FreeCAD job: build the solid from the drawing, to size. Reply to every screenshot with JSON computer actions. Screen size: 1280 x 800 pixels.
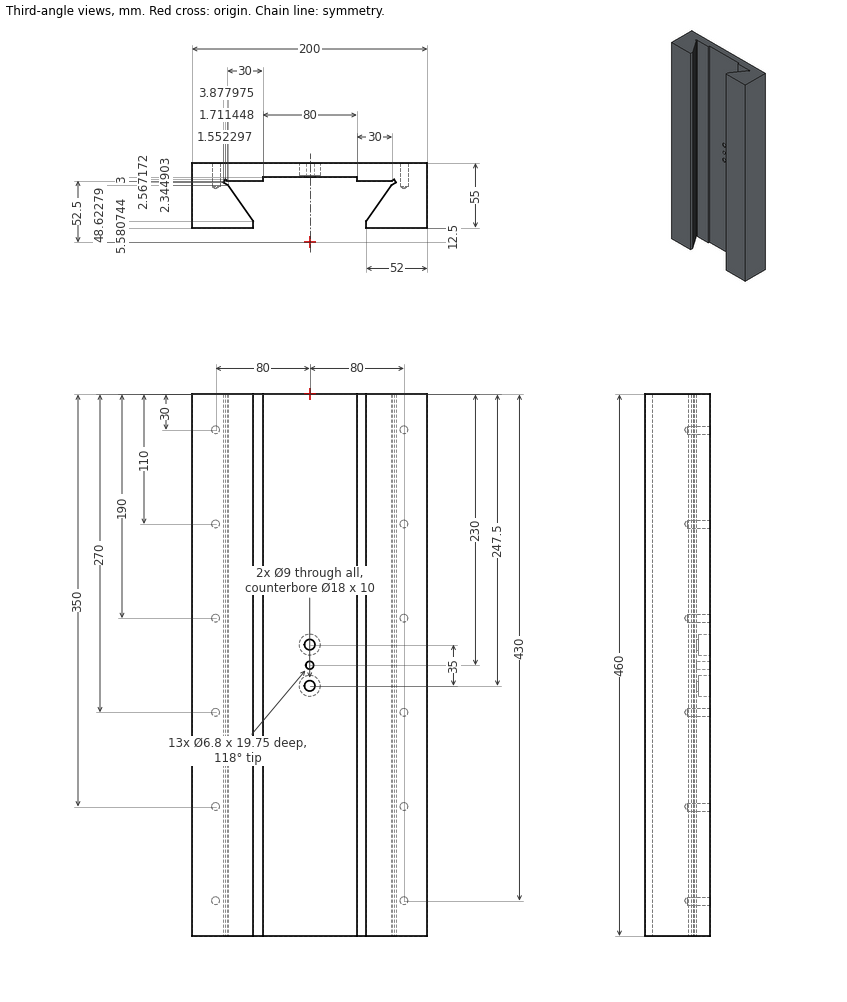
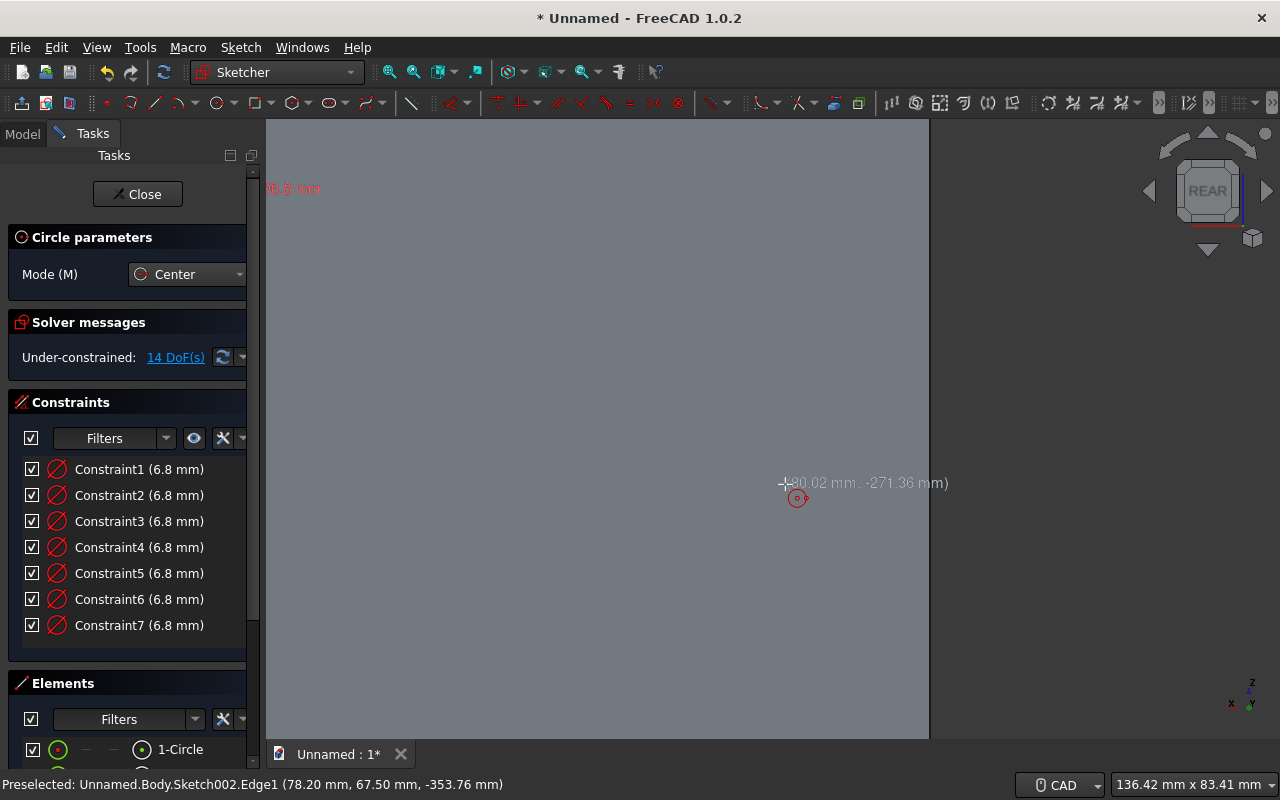
{"action": "scroll", "coordinate": [786, 483], "scroll_direction": "down", "scroll_amount": 10}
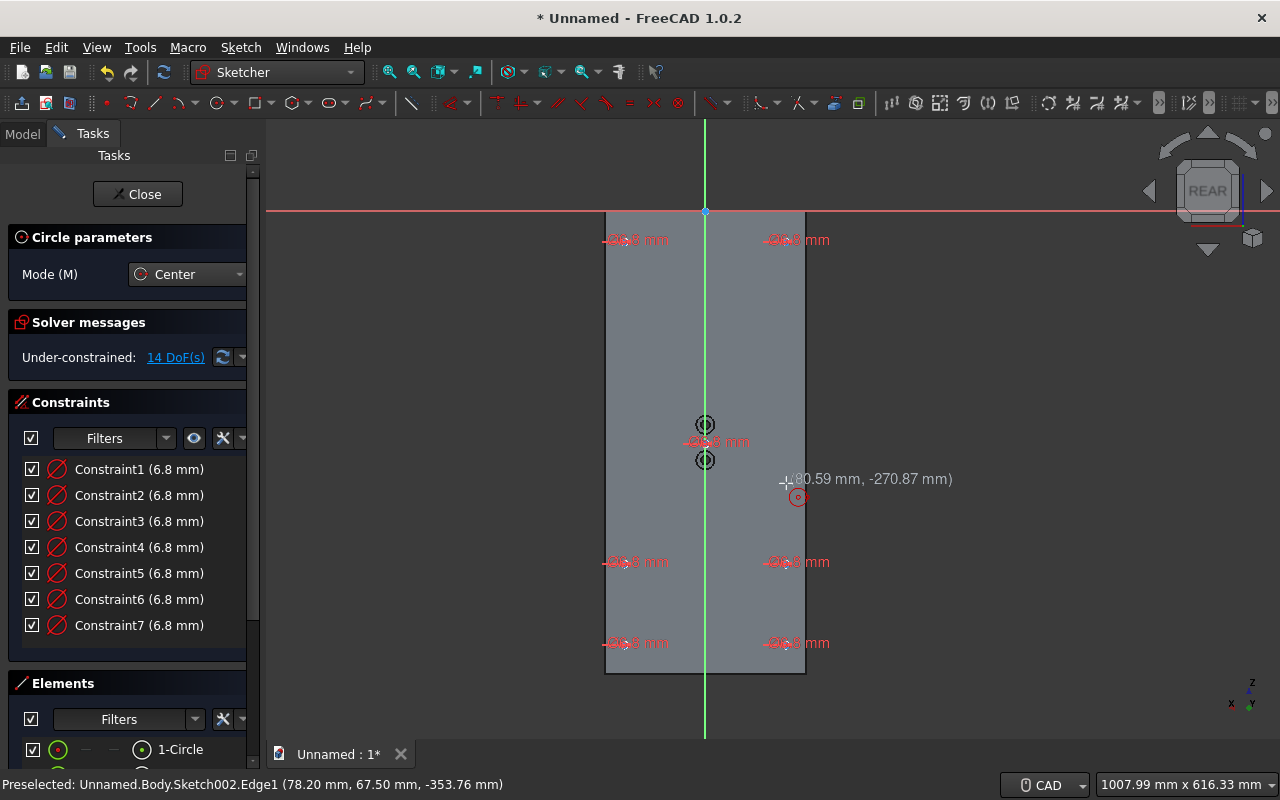
{"action": "left_click", "coordinate": [786, 483]}
{"action": "mouse_move", "coordinate": [788, 480]}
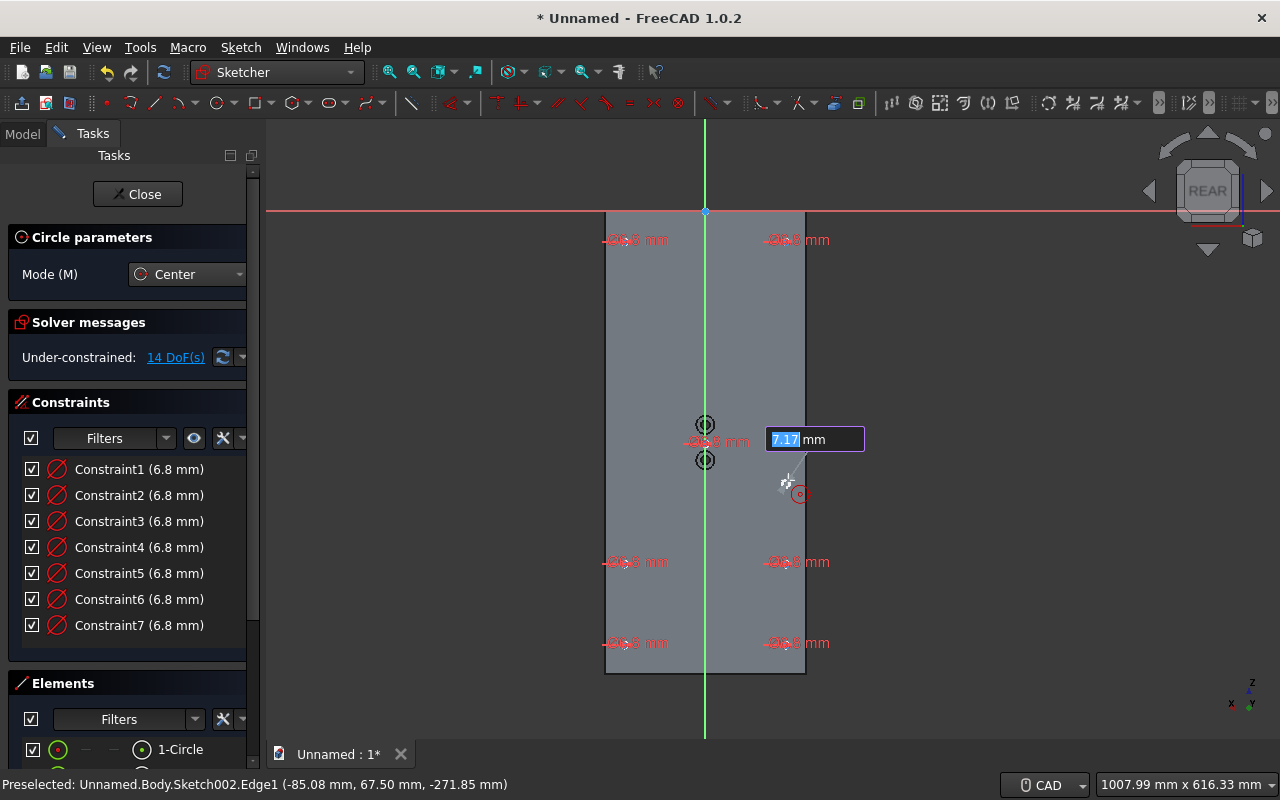
{"action": "type", "text": "6.8"}
{"action": "key", "text": "Return"}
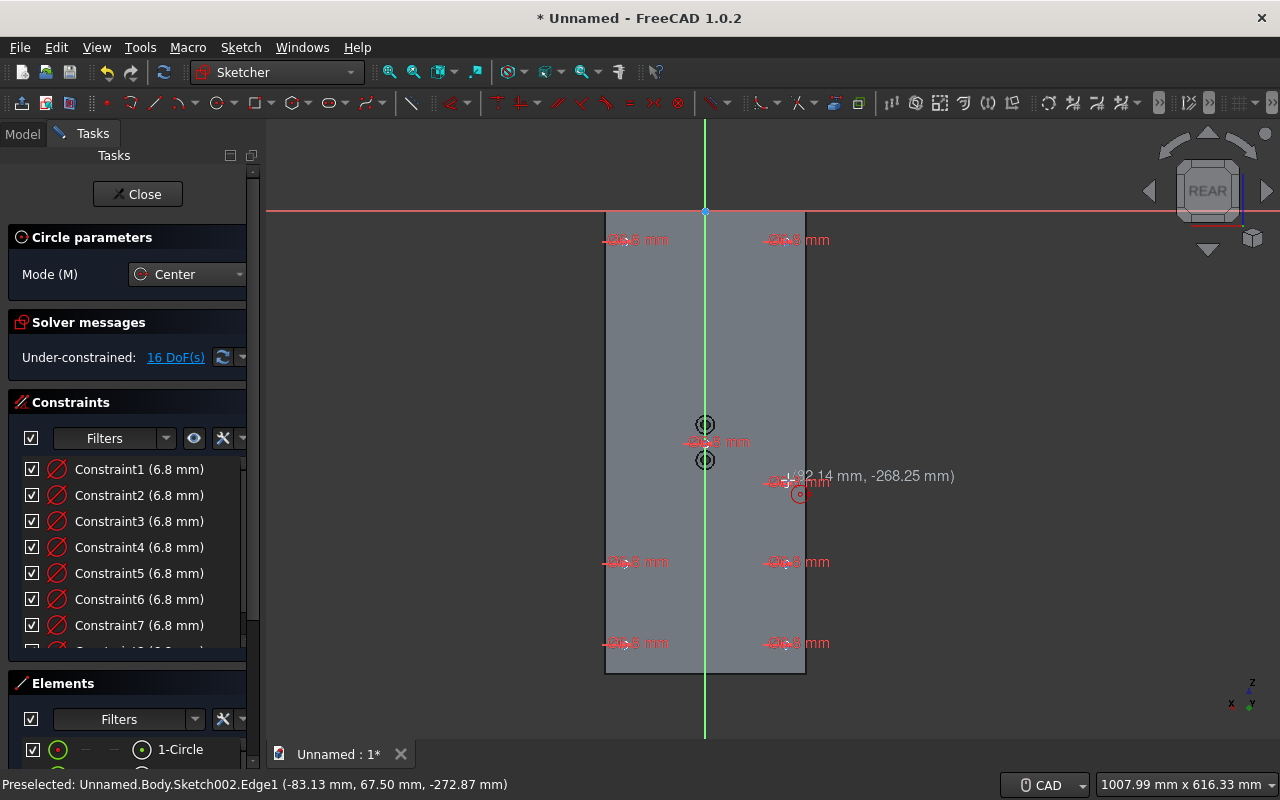
{"action": "scroll", "coordinate": [625, 483], "scroll_direction": "up", "scroll_amount": 10}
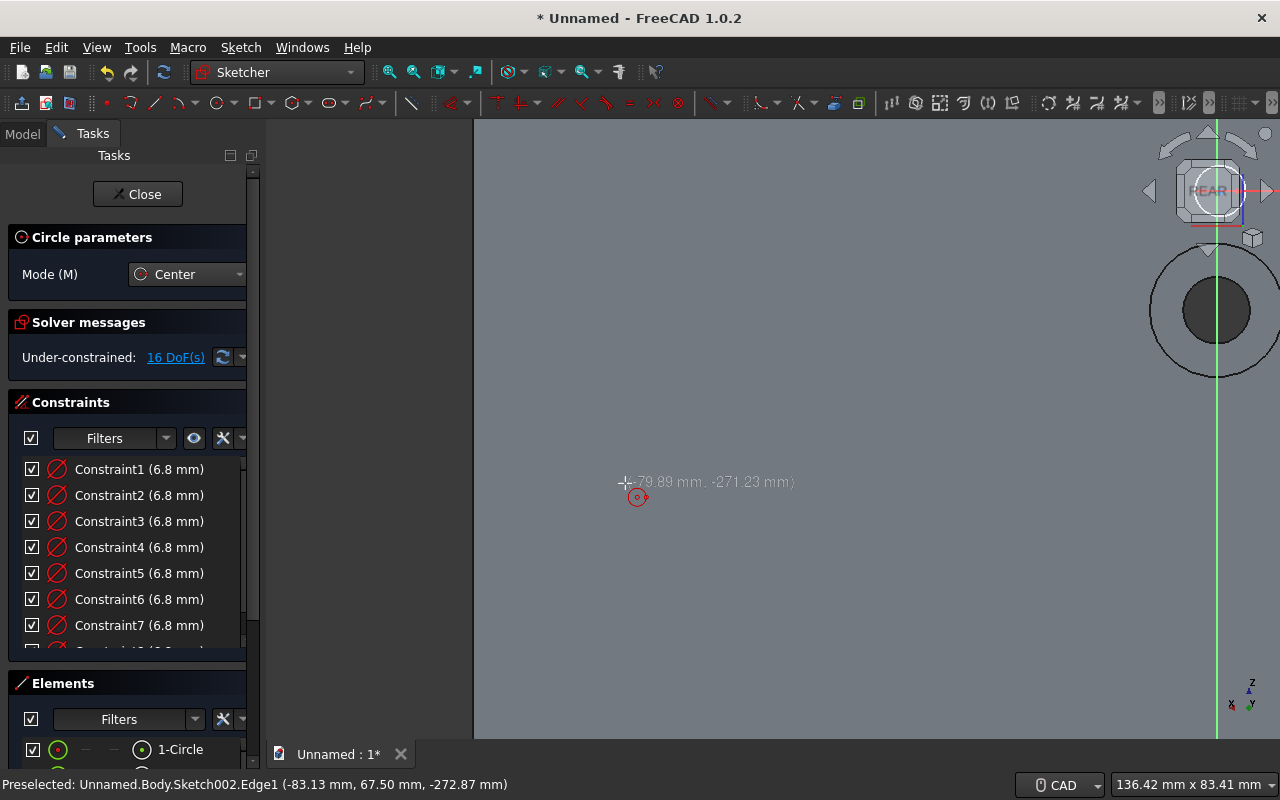
{"action": "scroll", "coordinate": [624, 483], "scroll_direction": "down", "scroll_amount": 10}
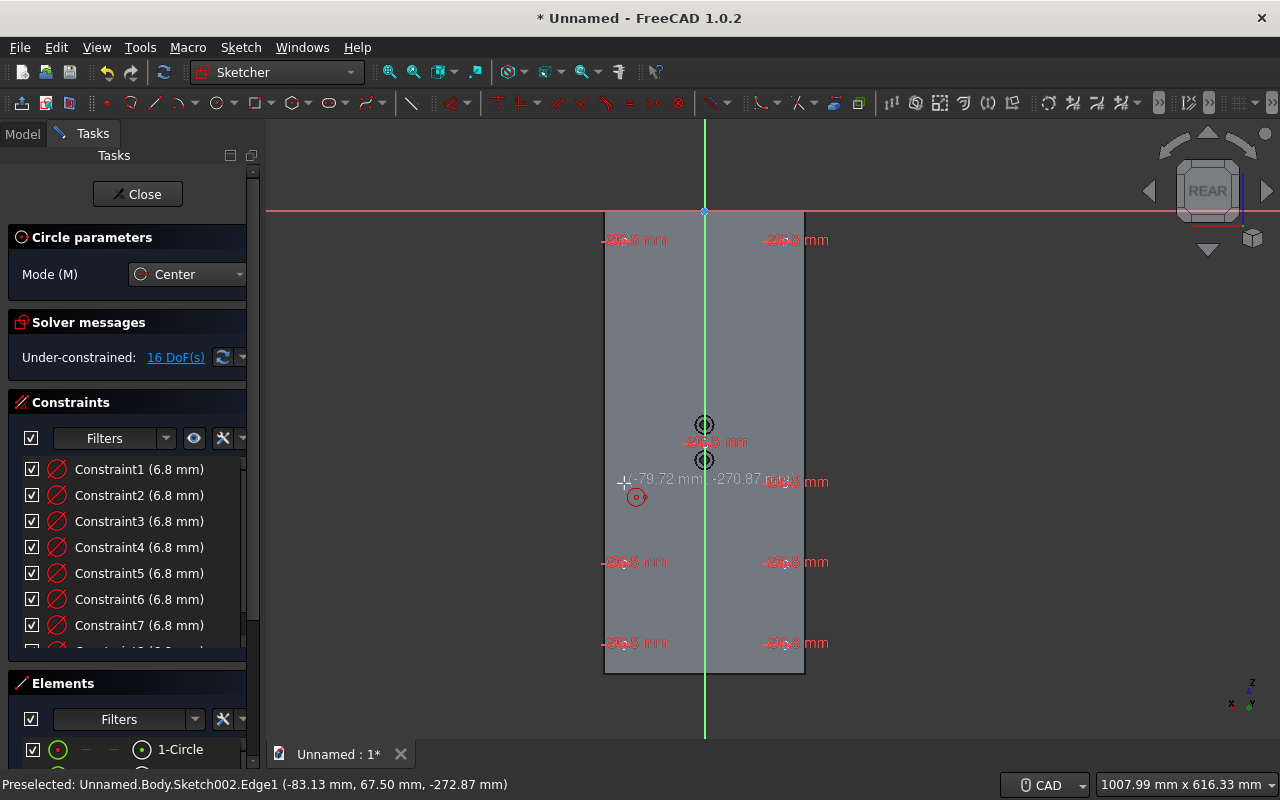
{"action": "left_click", "coordinate": [624, 483]}
{"action": "mouse_move", "coordinate": [626, 480]}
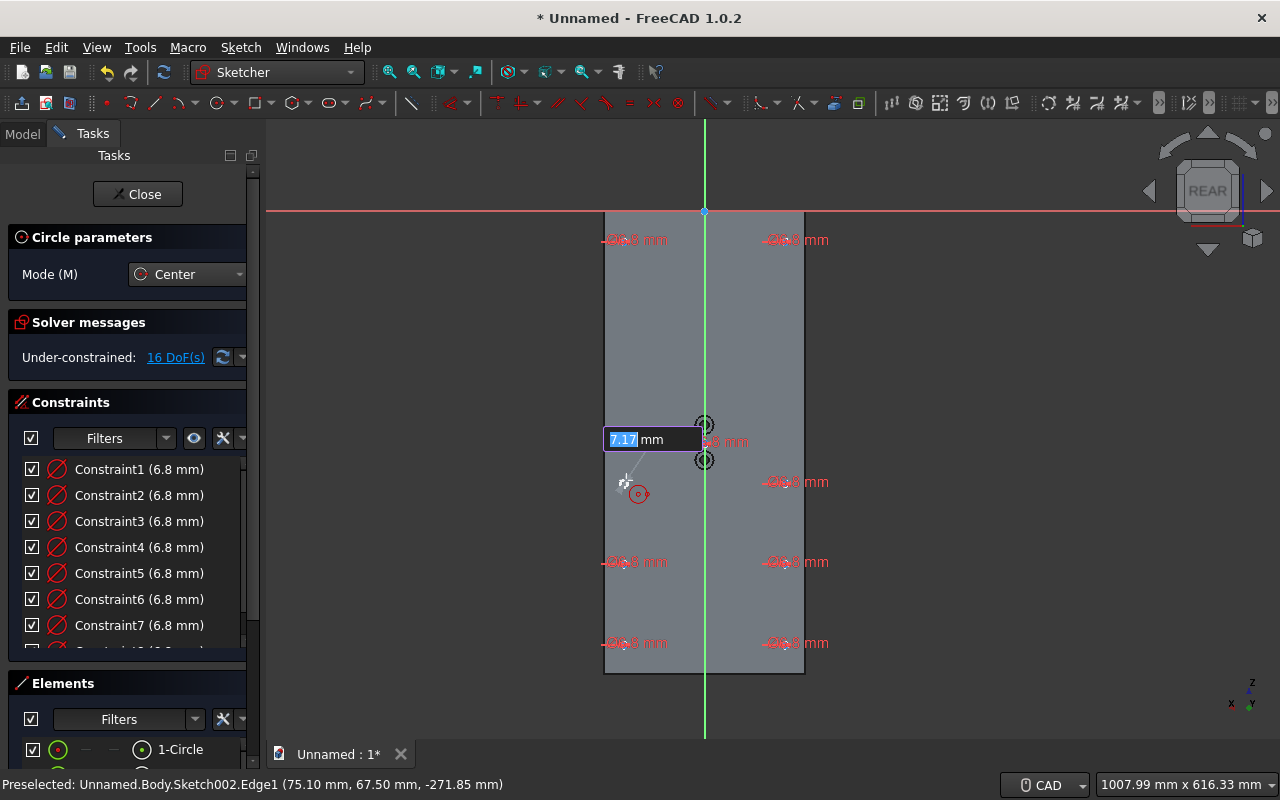
{"action": "type", "text": "6.8"}
{"action": "key", "text": "Return"}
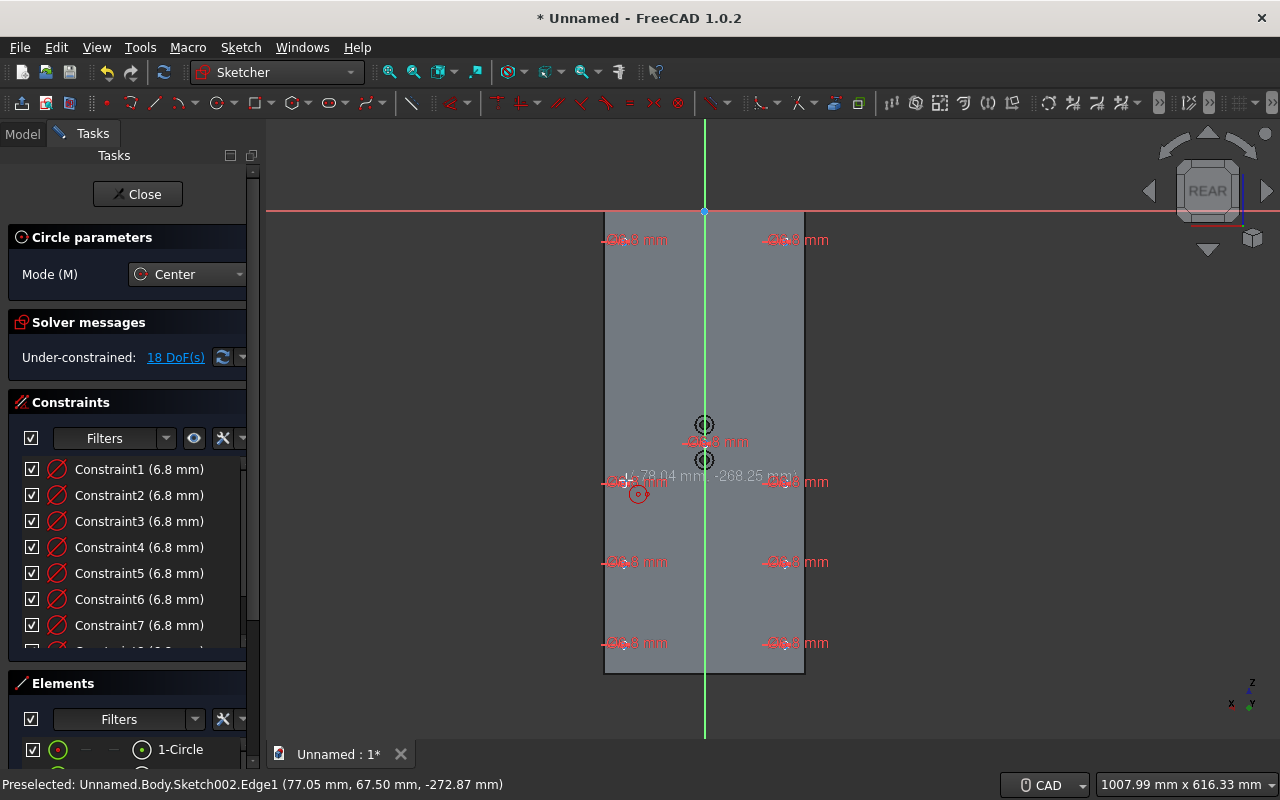
{"action": "scroll", "coordinate": [785, 402], "scroll_direction": "up", "scroll_amount": 10}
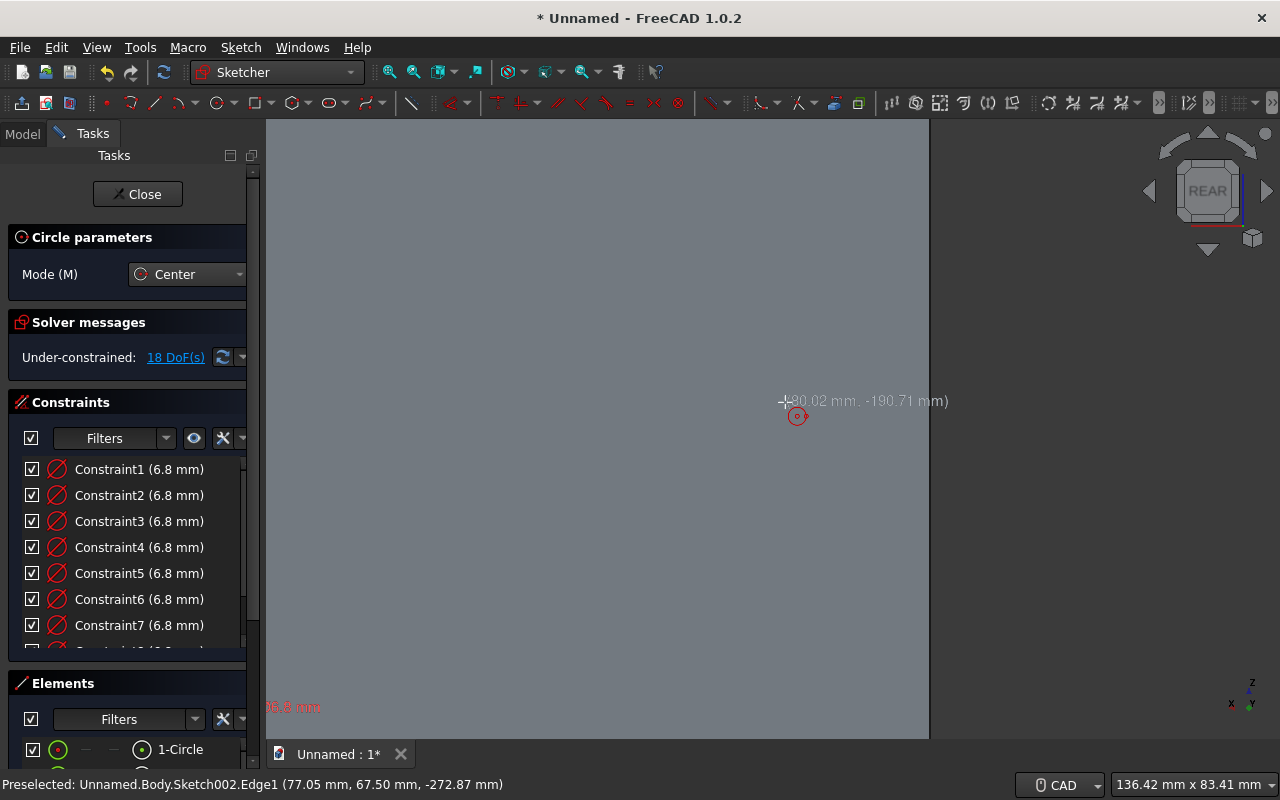
{"action": "scroll", "coordinate": [786, 402], "scroll_direction": "down", "scroll_amount": 10}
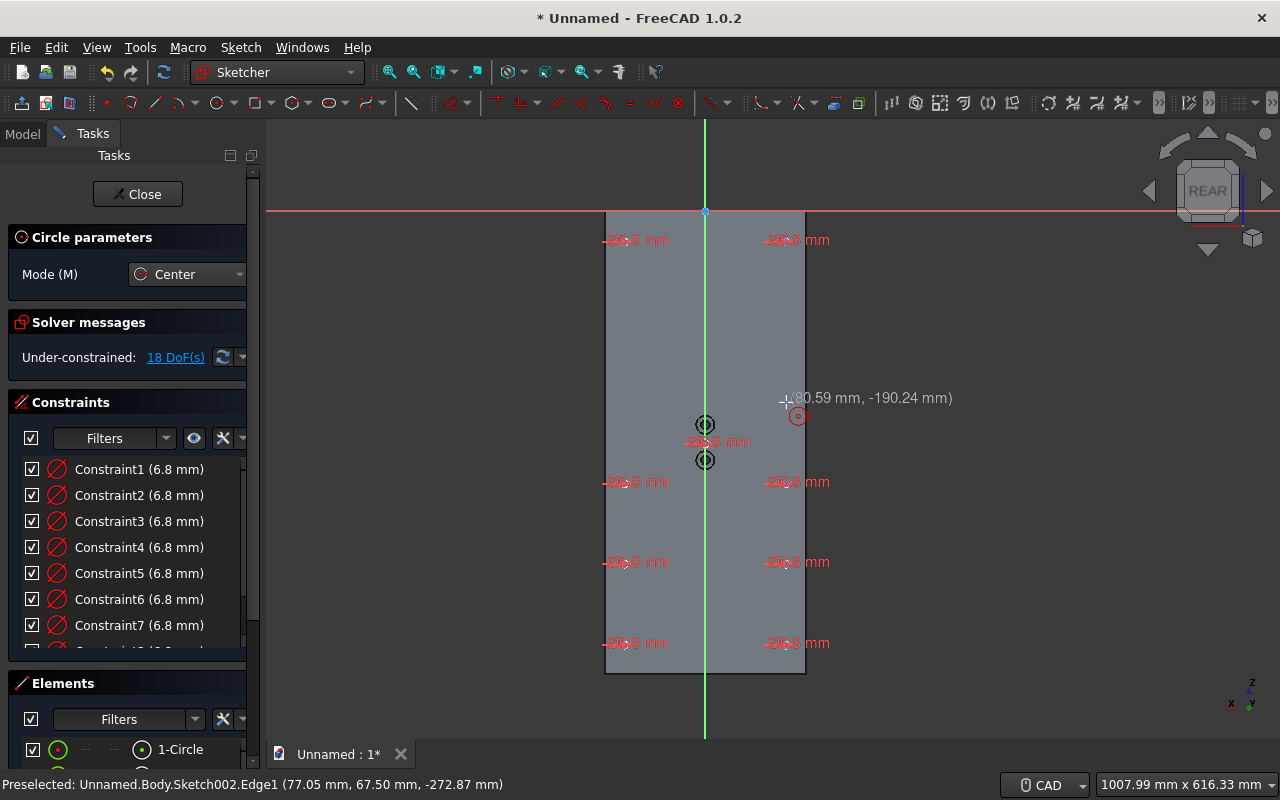
{"action": "left_click", "coordinate": [786, 402]}
{"action": "mouse_move", "coordinate": [788, 400]}